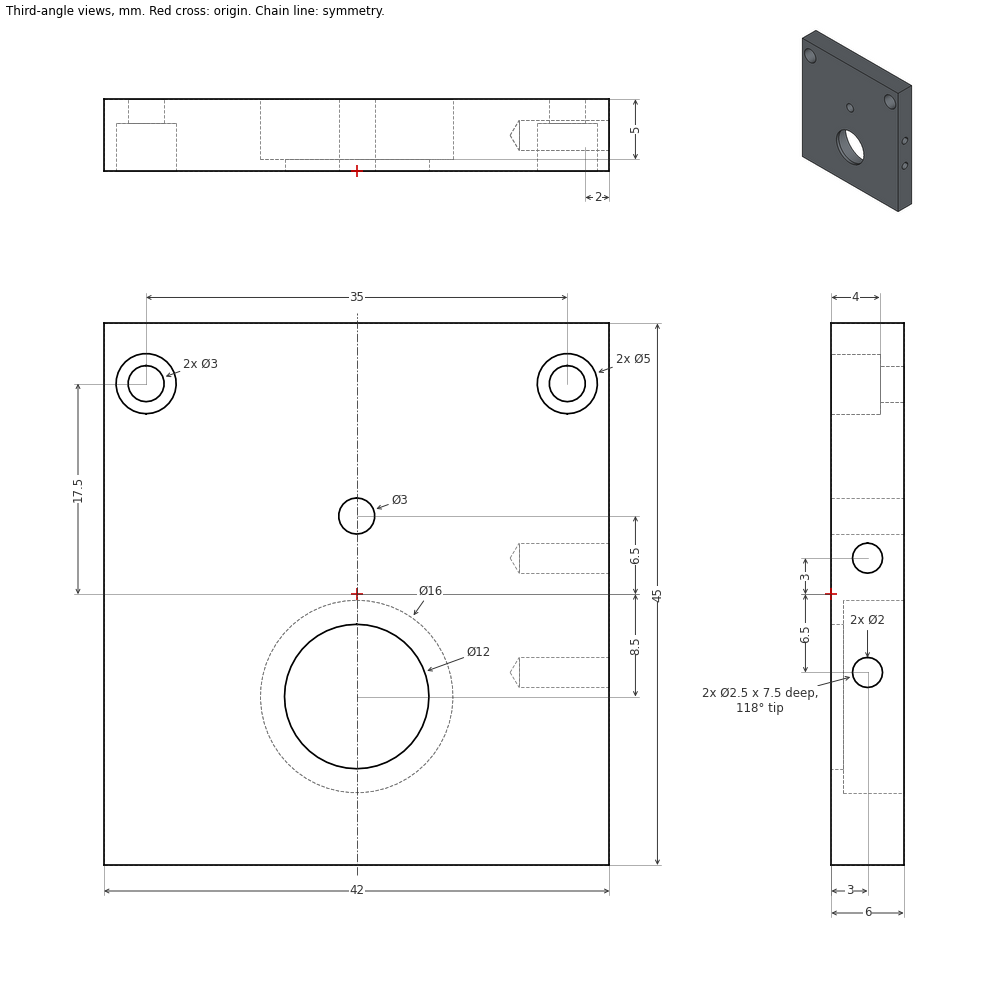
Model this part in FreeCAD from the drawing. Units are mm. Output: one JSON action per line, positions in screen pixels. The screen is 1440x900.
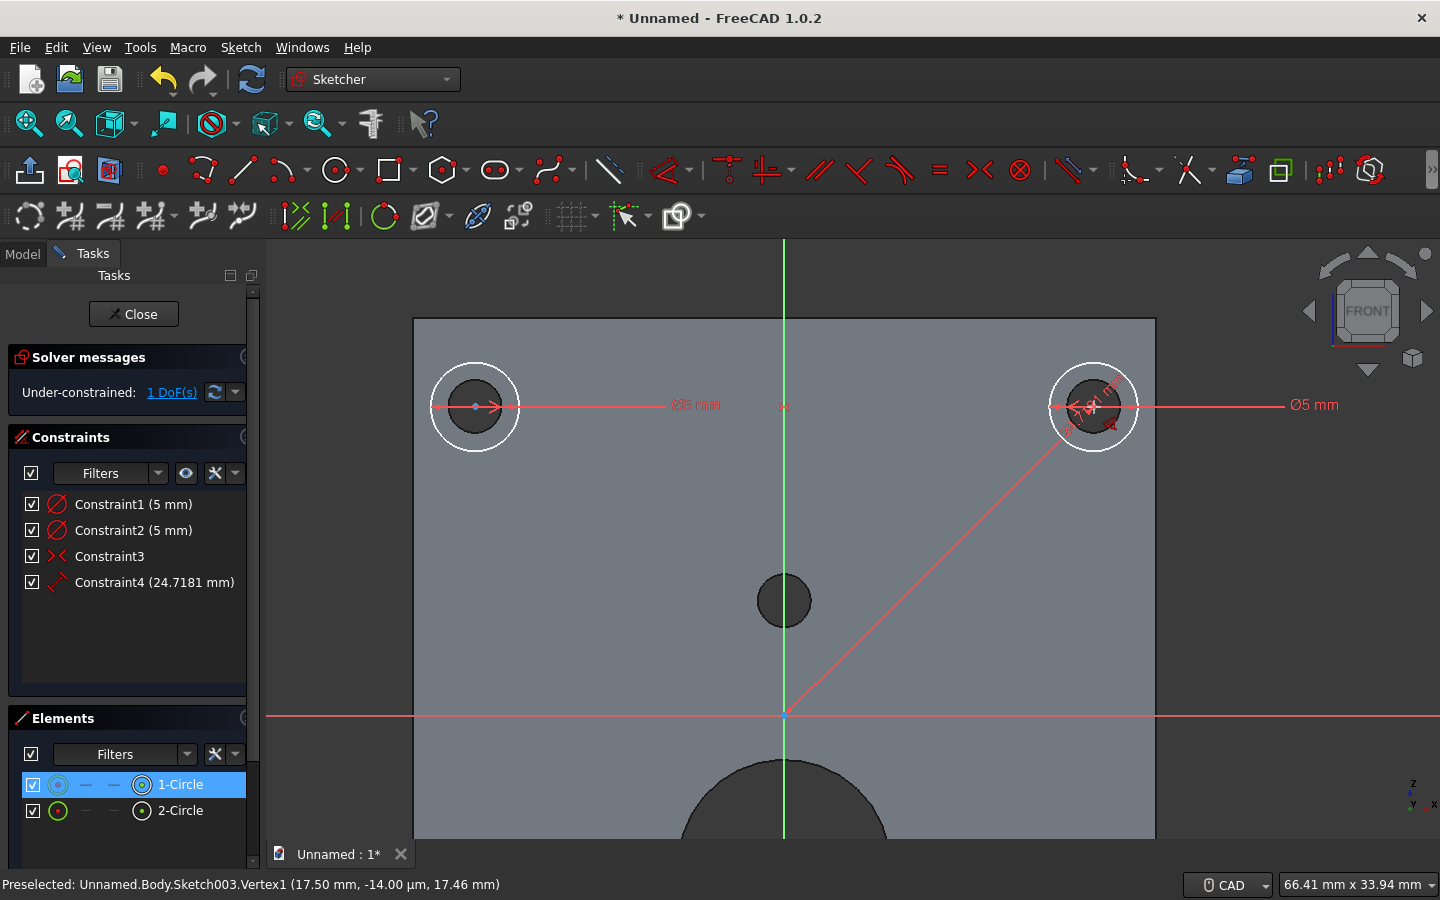
{"action": "left_click", "coordinate": [475, 407]}
{"action": "left_click", "coordinate": [642, 373]}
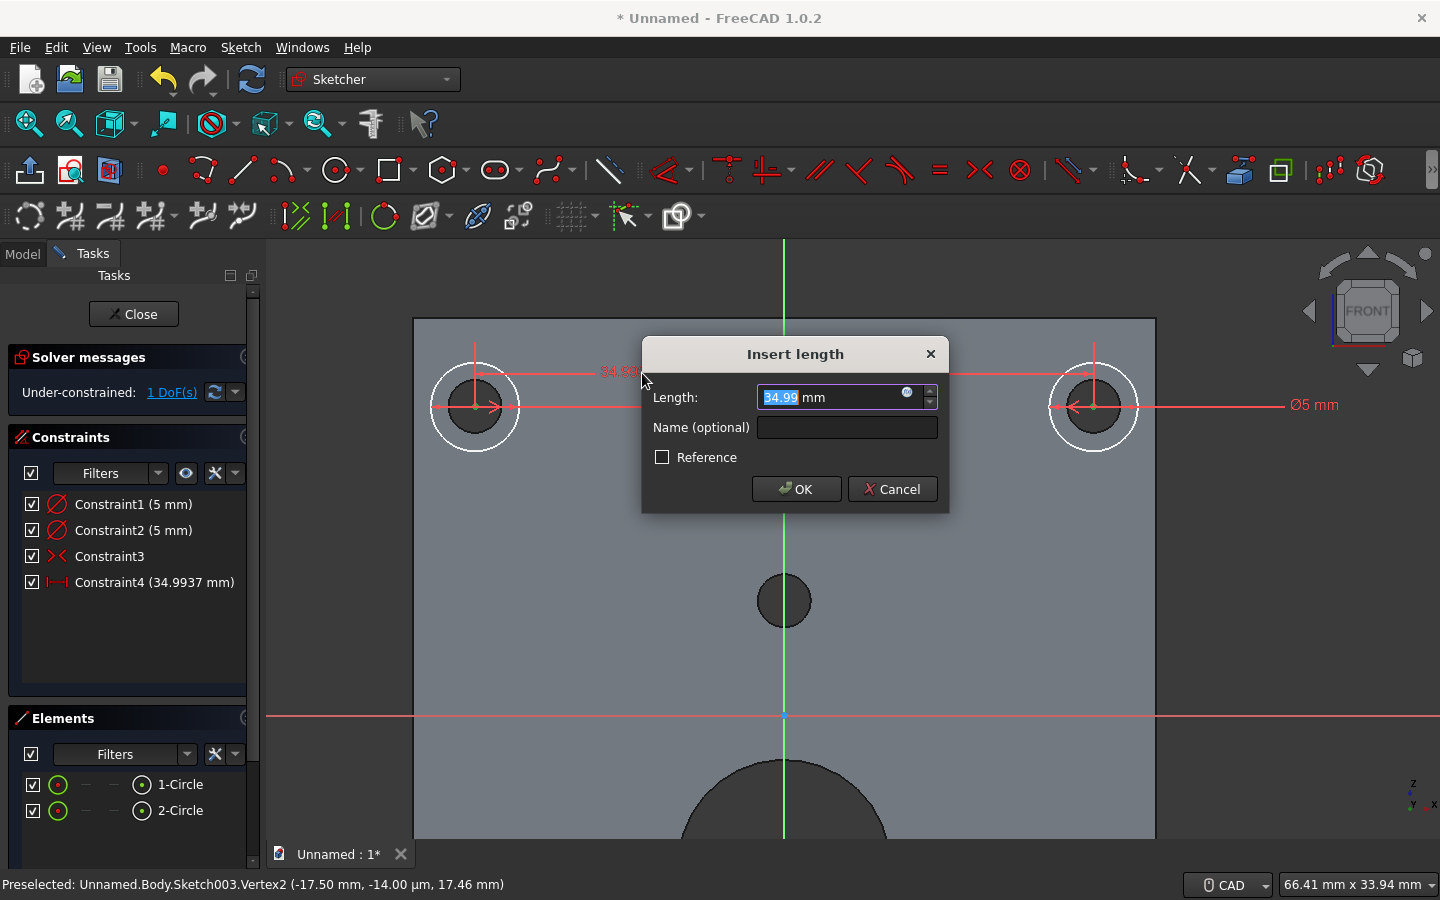
{"action": "type", "text": "35"}
{"action": "key", "text": "Return"}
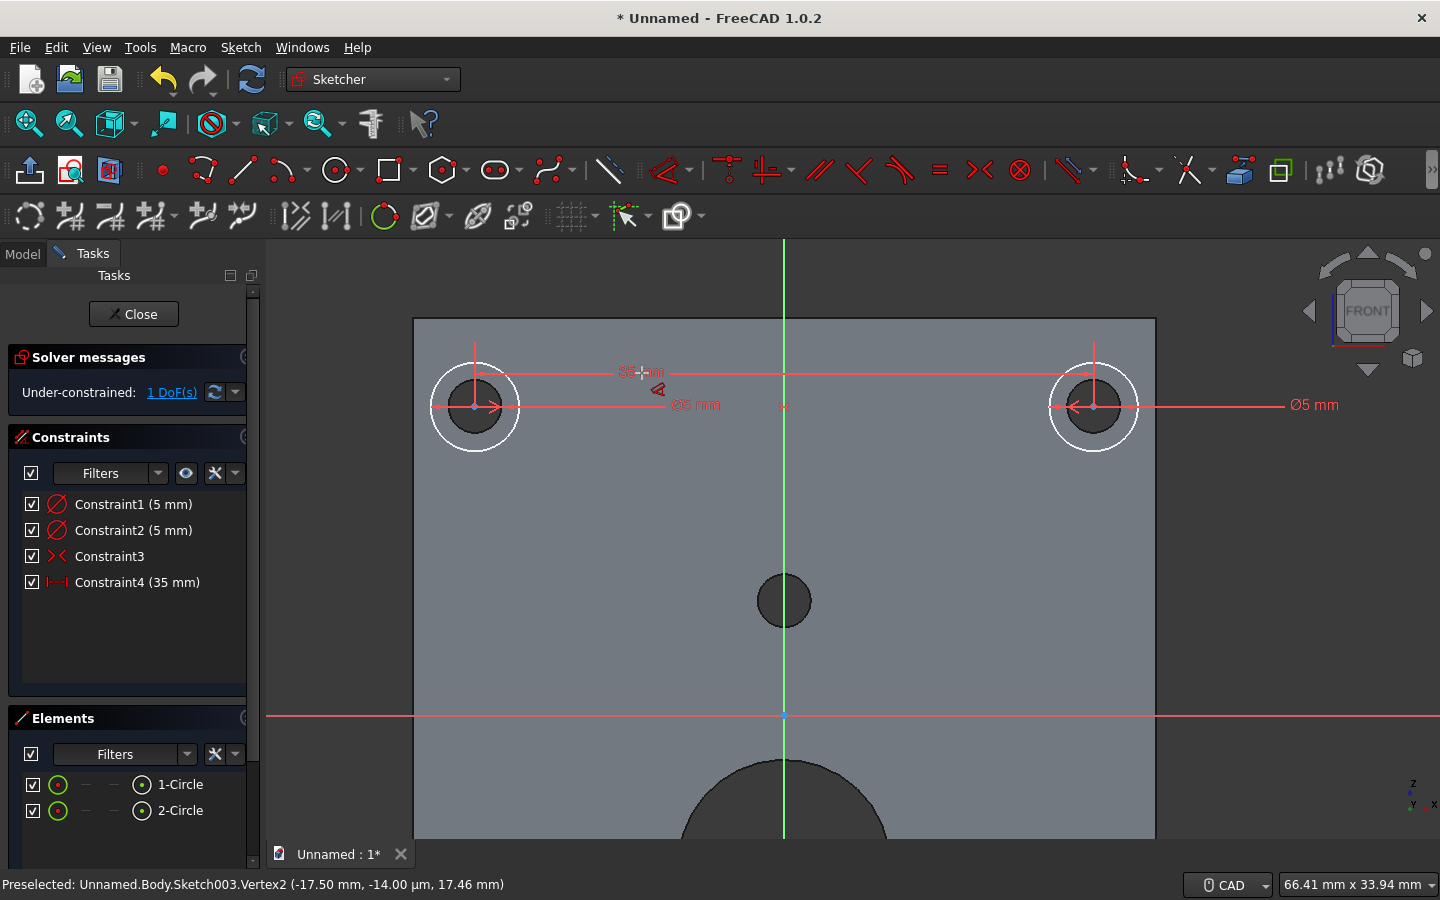
{"action": "left_click", "coordinate": [1094, 407]}
{"action": "left_click", "coordinate": [1128, 561]}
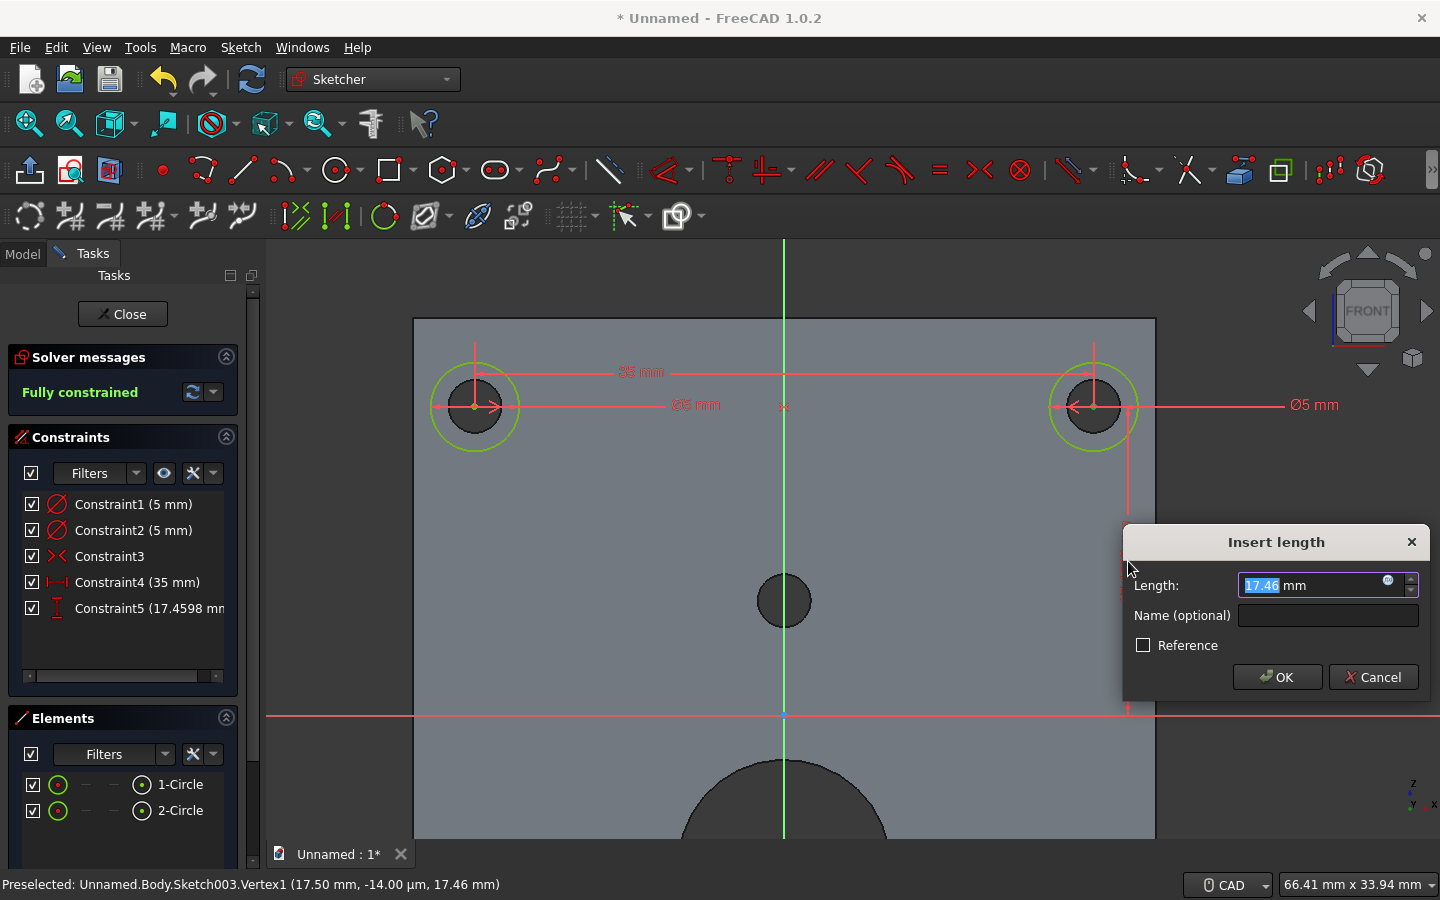
{"action": "type", "text": "17.5"}
{"action": "key", "text": "Return"}
{"action": "key", "text": "Escape"}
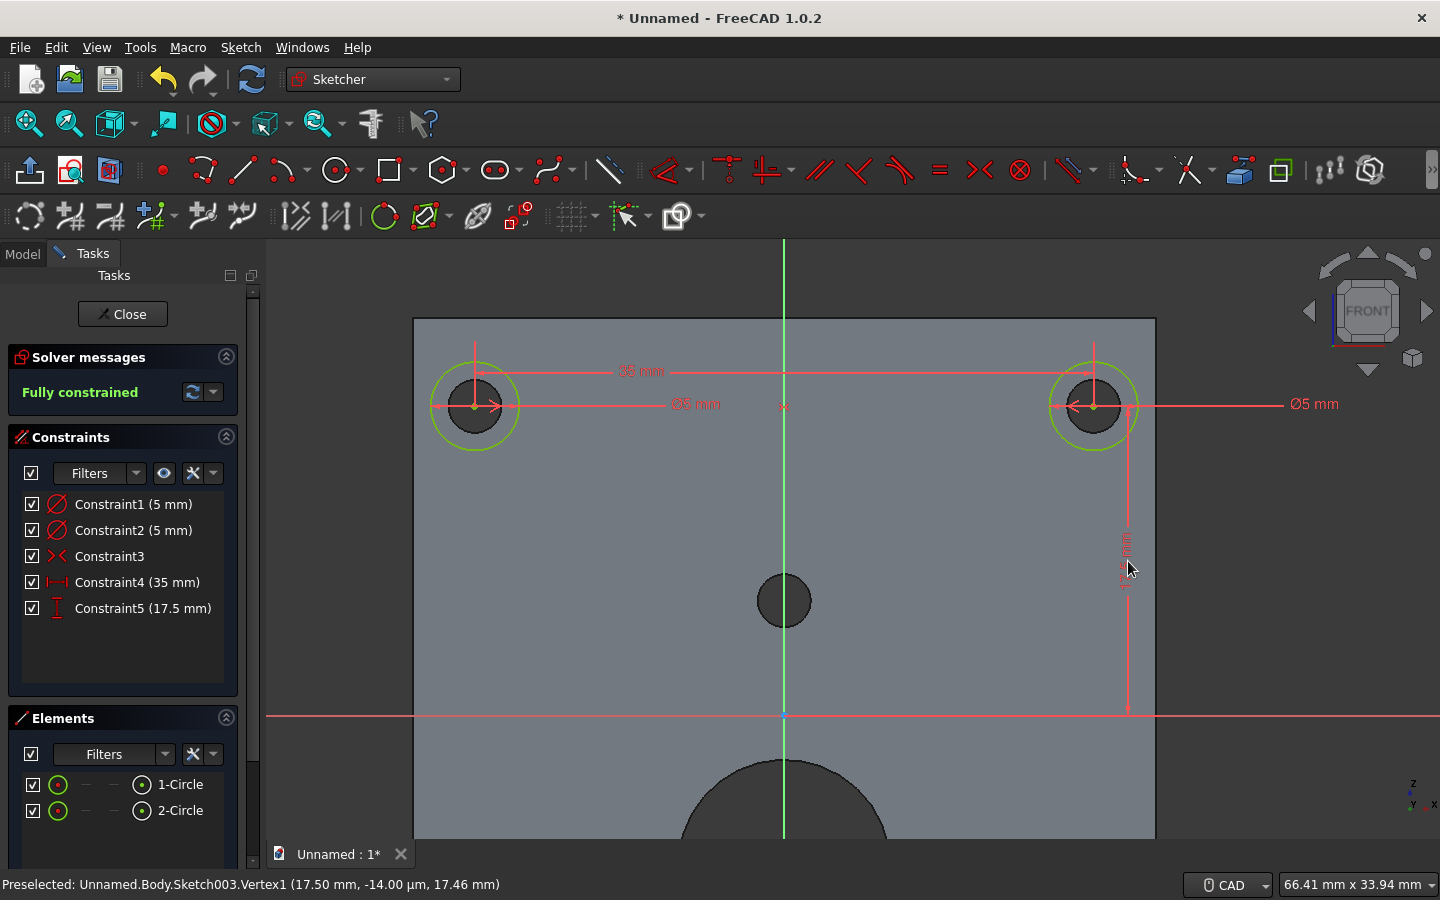
{"action": "left_click", "coordinate": [123, 314]}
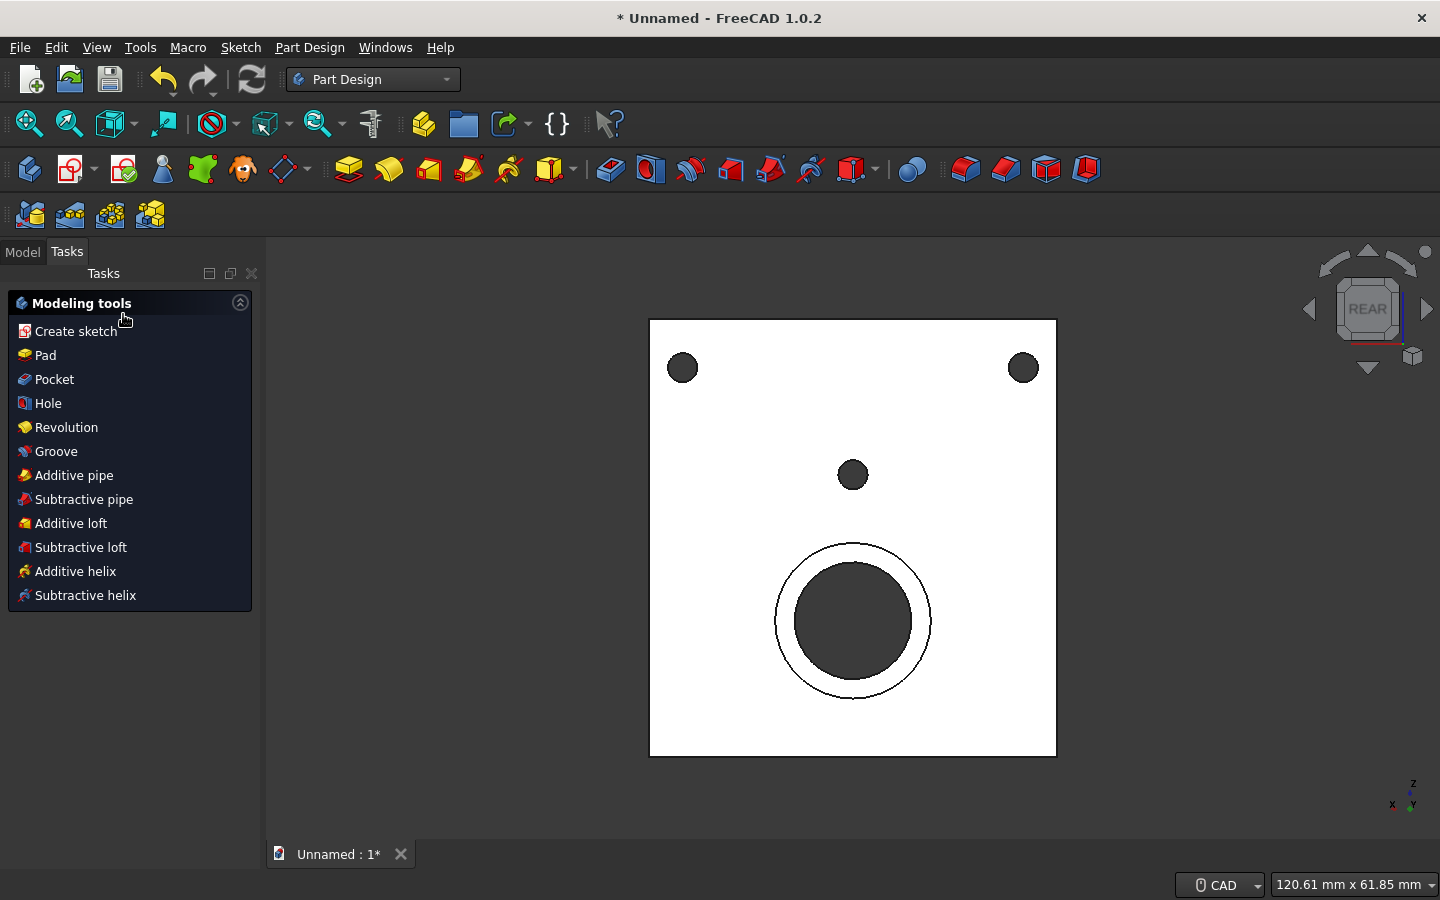
{"action": "left_click", "coordinate": [612, 170]}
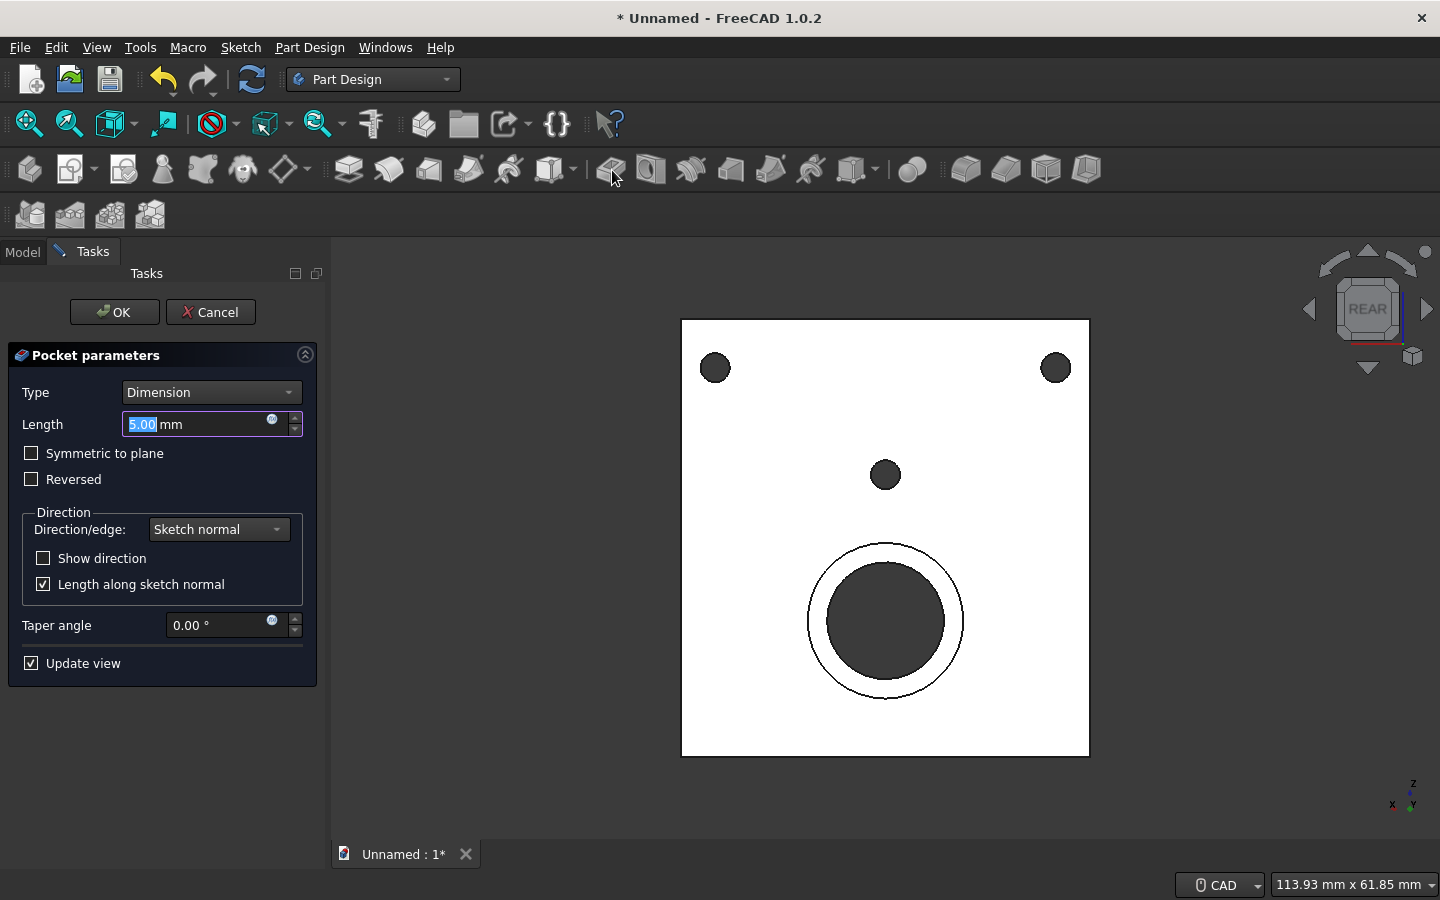
{"action": "type", "text": "4"}
{"action": "key", "text": "Tab"}